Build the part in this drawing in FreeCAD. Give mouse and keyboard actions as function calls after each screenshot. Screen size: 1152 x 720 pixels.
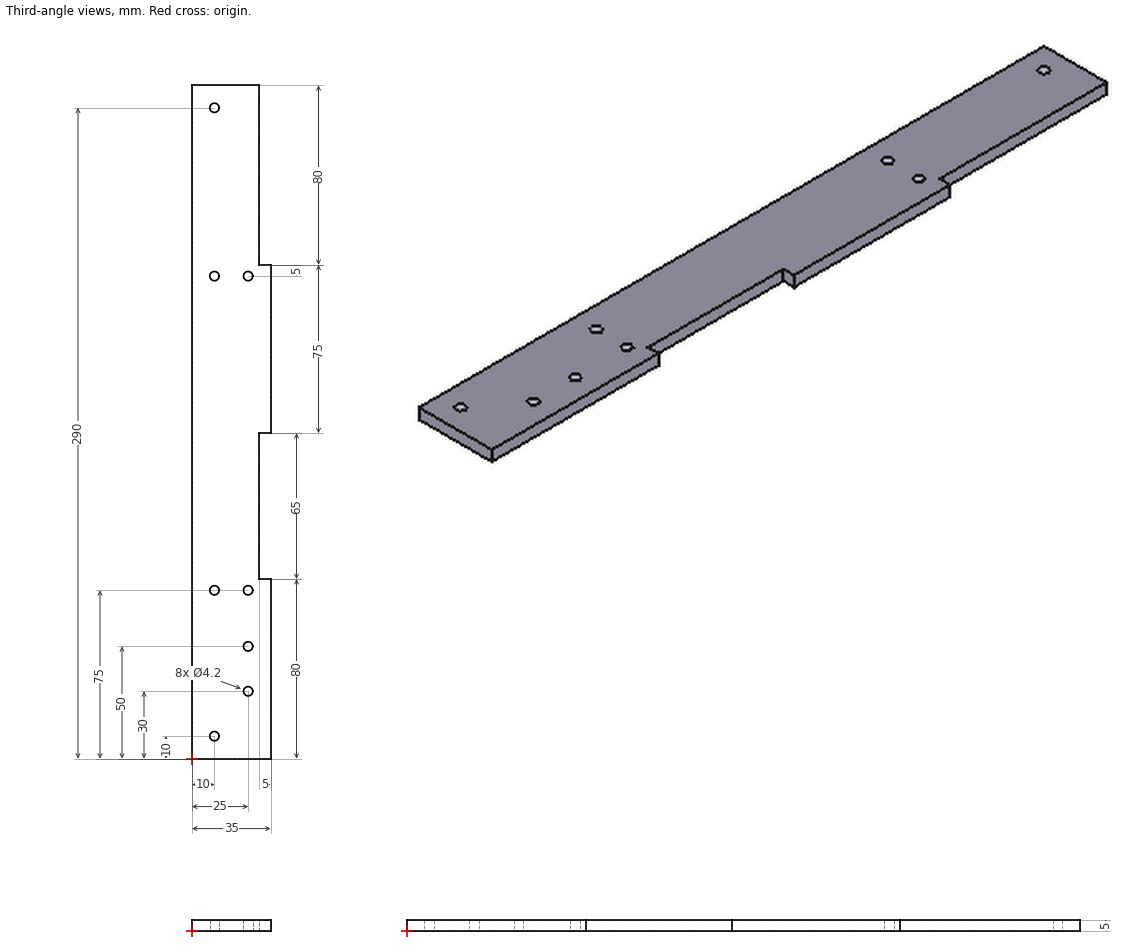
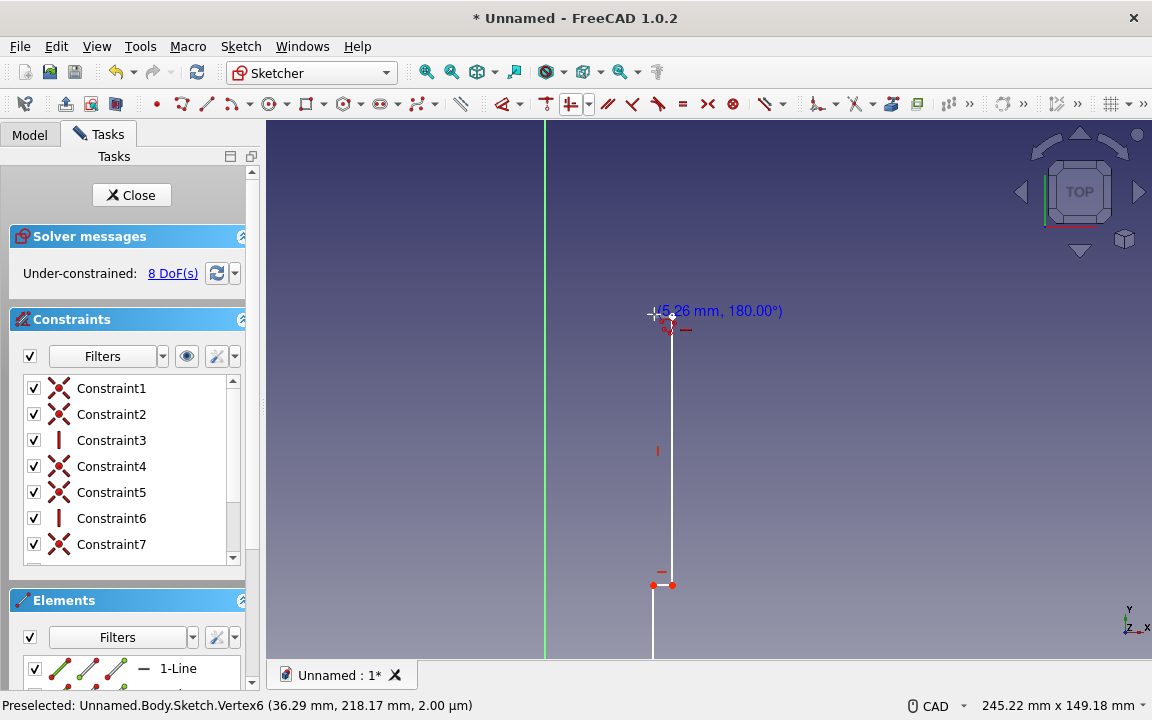
click(653, 313)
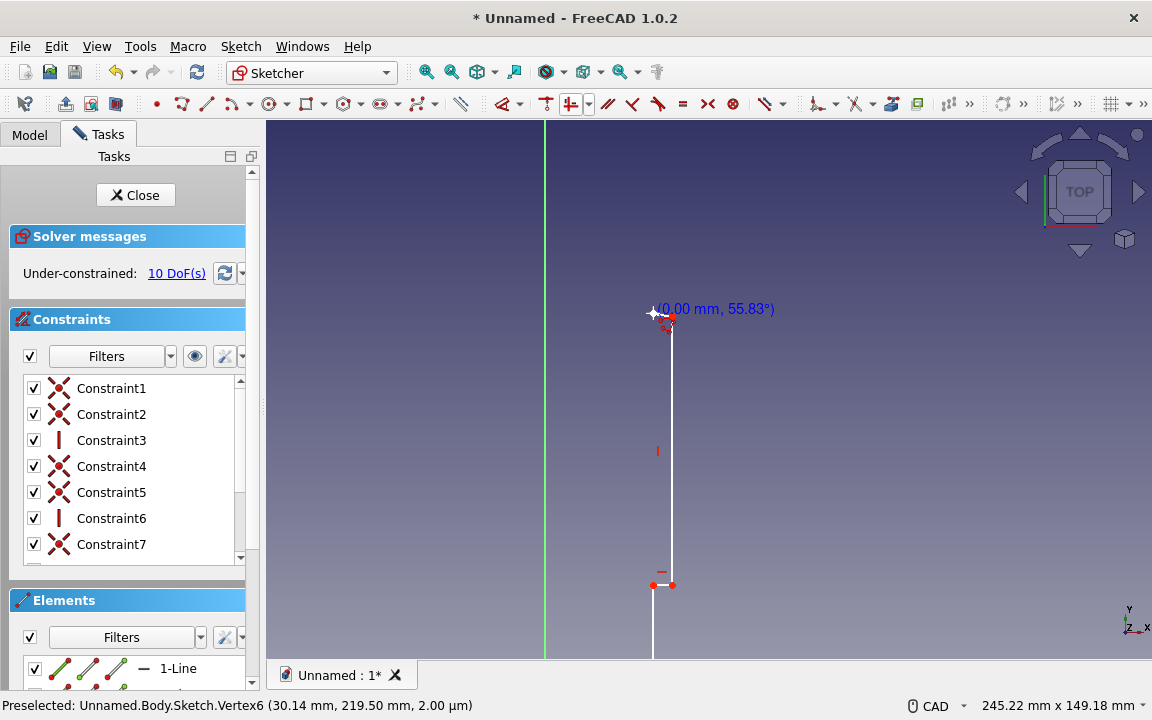
scroll(654, 313, down, 6)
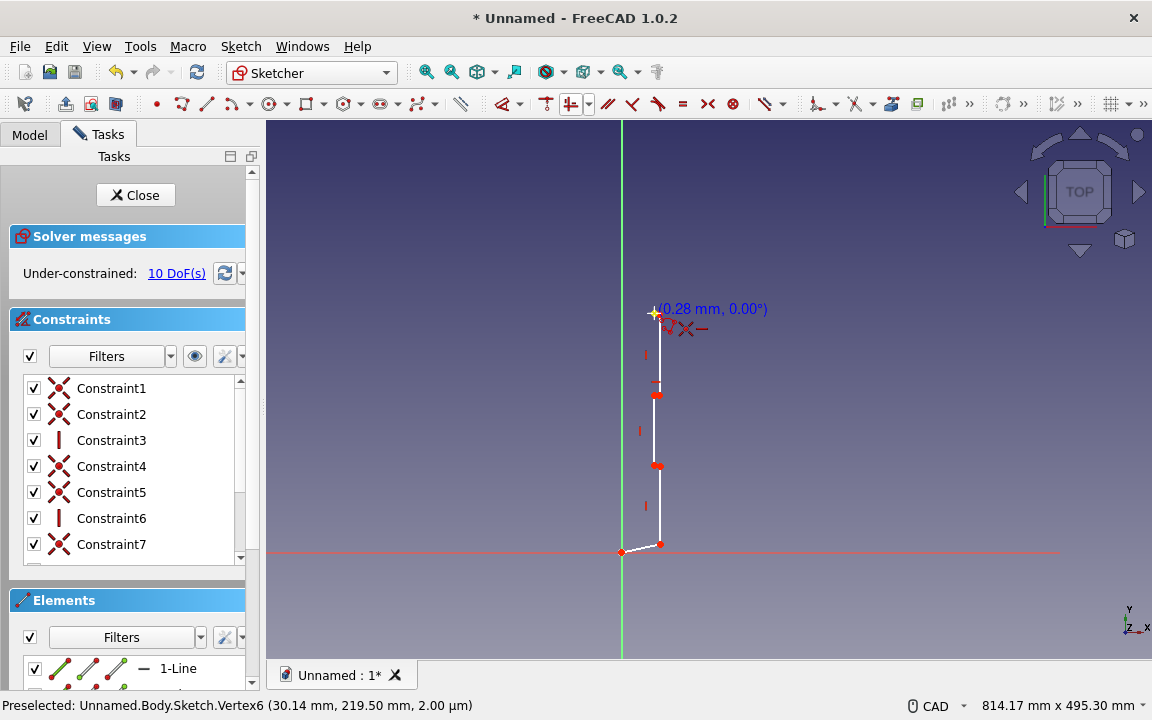
click(654, 226)
click(631, 226)
click(622, 553)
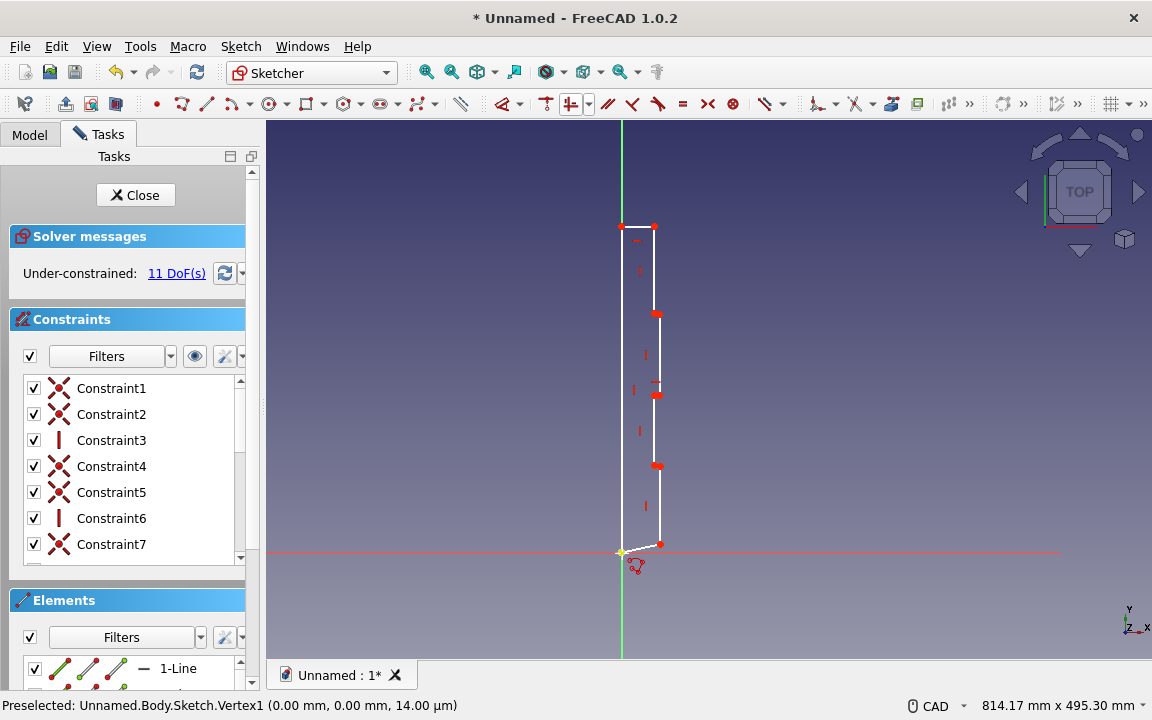
click(268, 104)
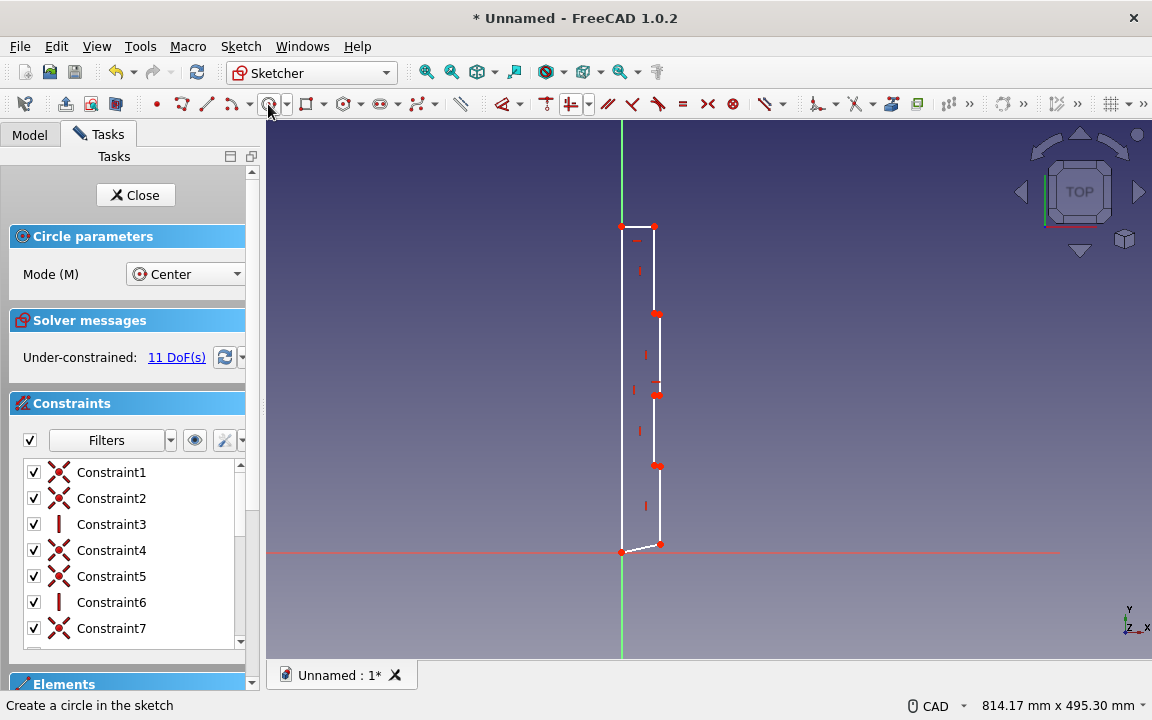
scroll(649, 520, up, 12)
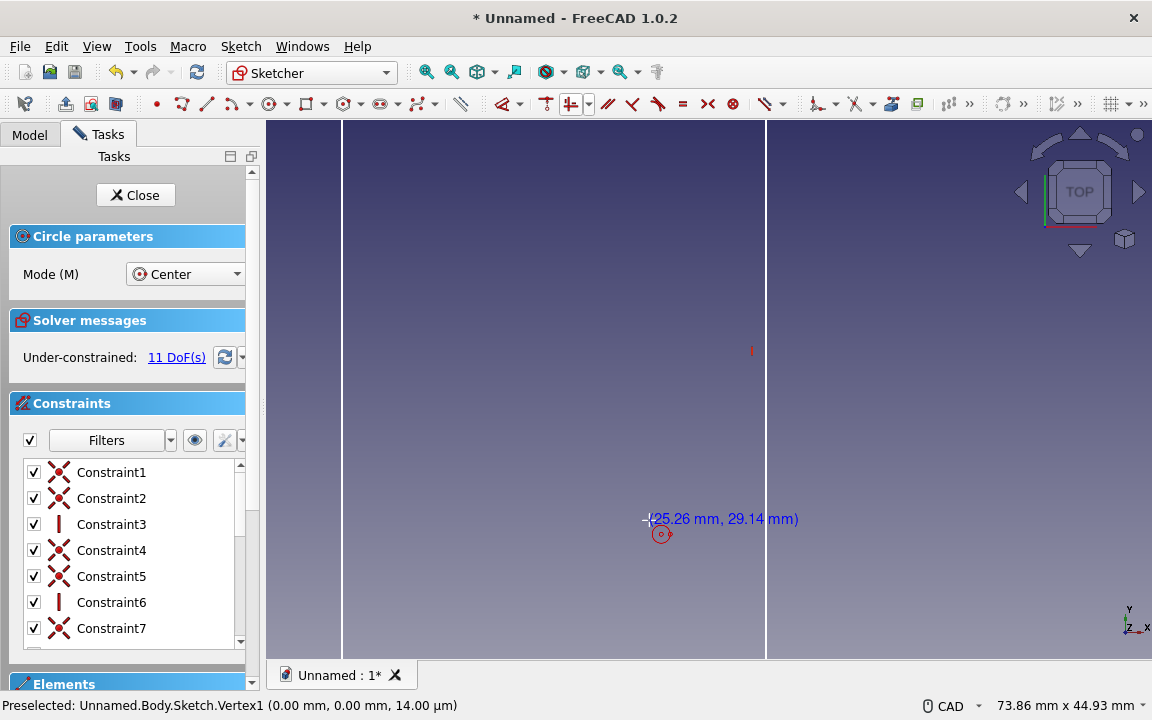
scroll(649, 521, down, 12)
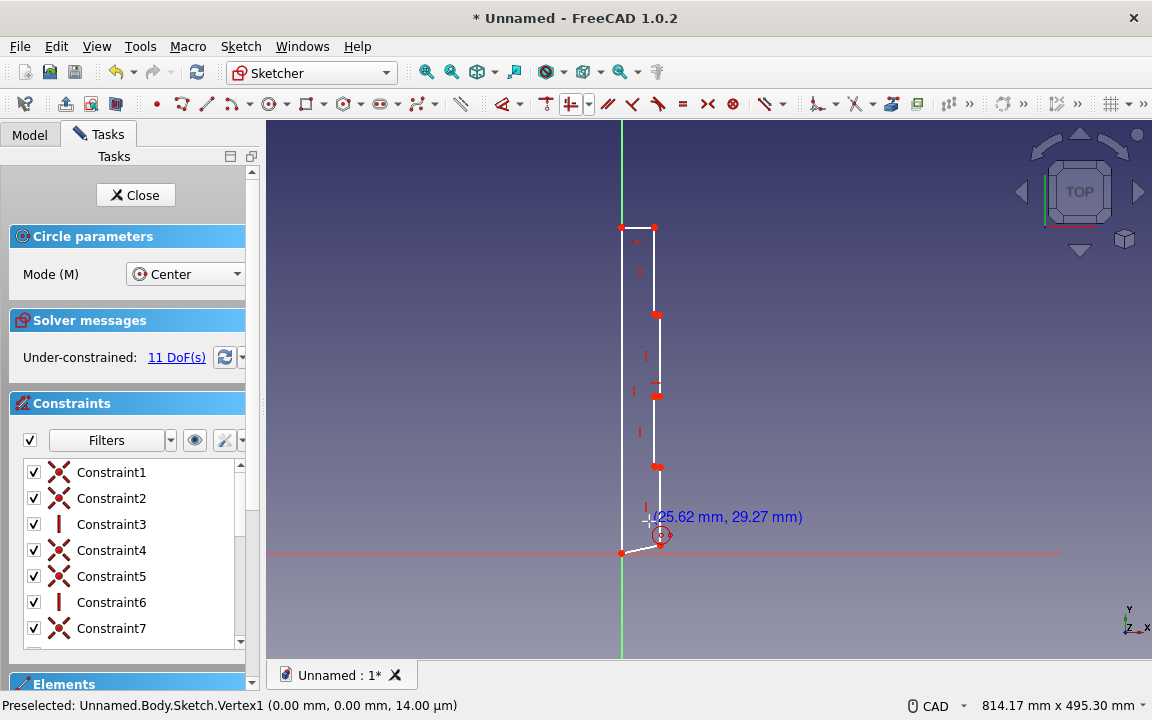
scroll(649, 521, up, 2)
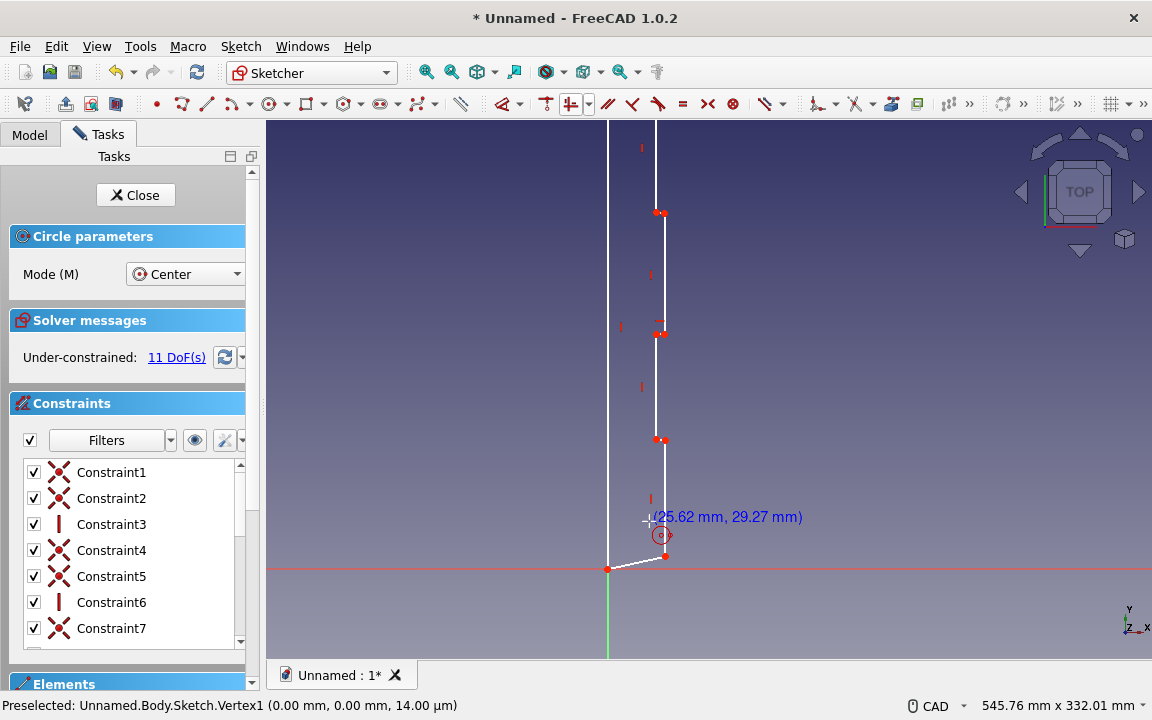
click(648, 521)
move(646, 518)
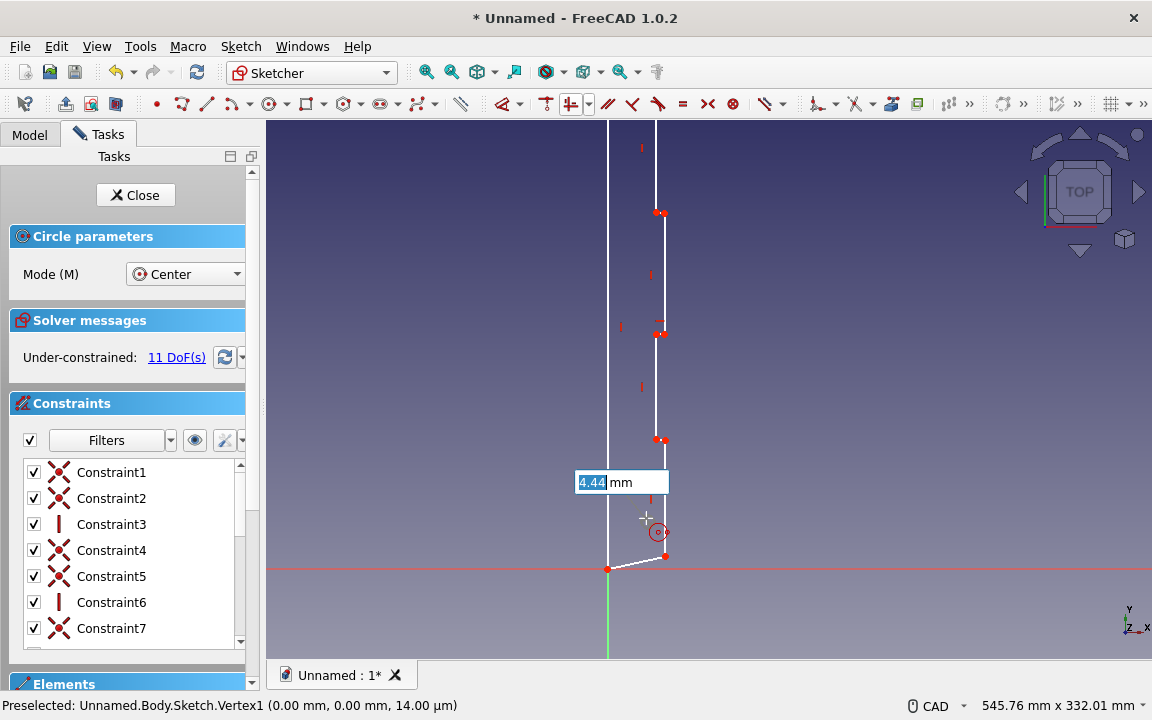
text(4.2)
key(Return)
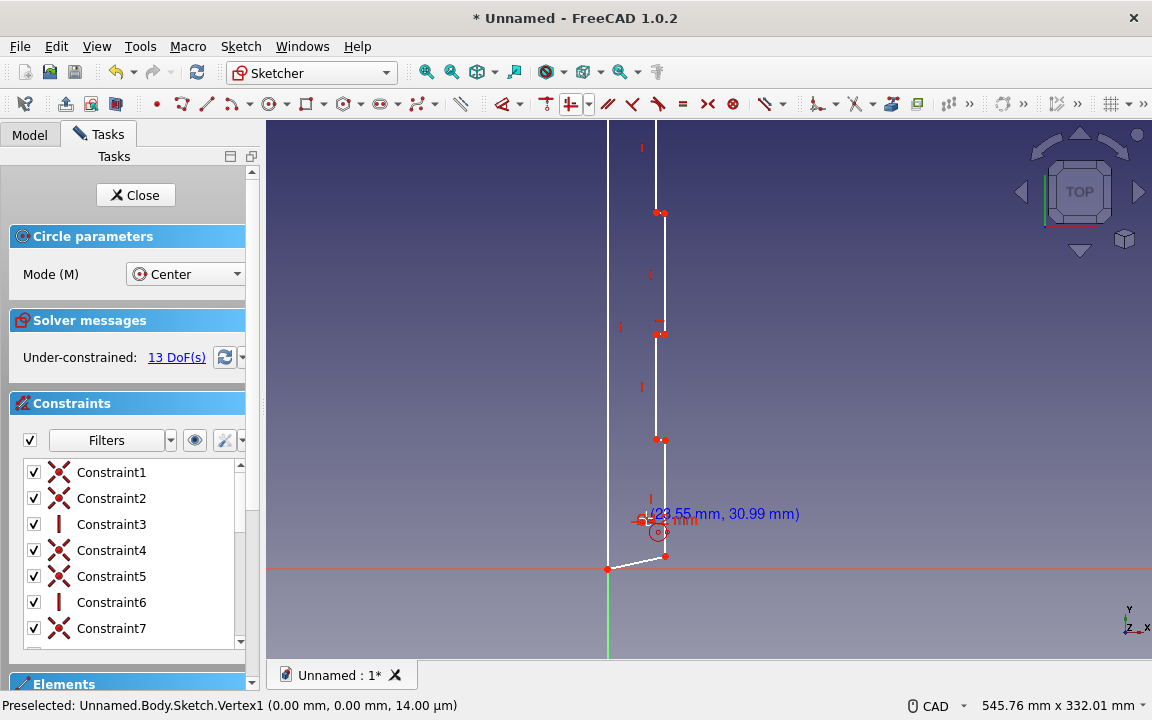
scroll(648, 488, up, 10)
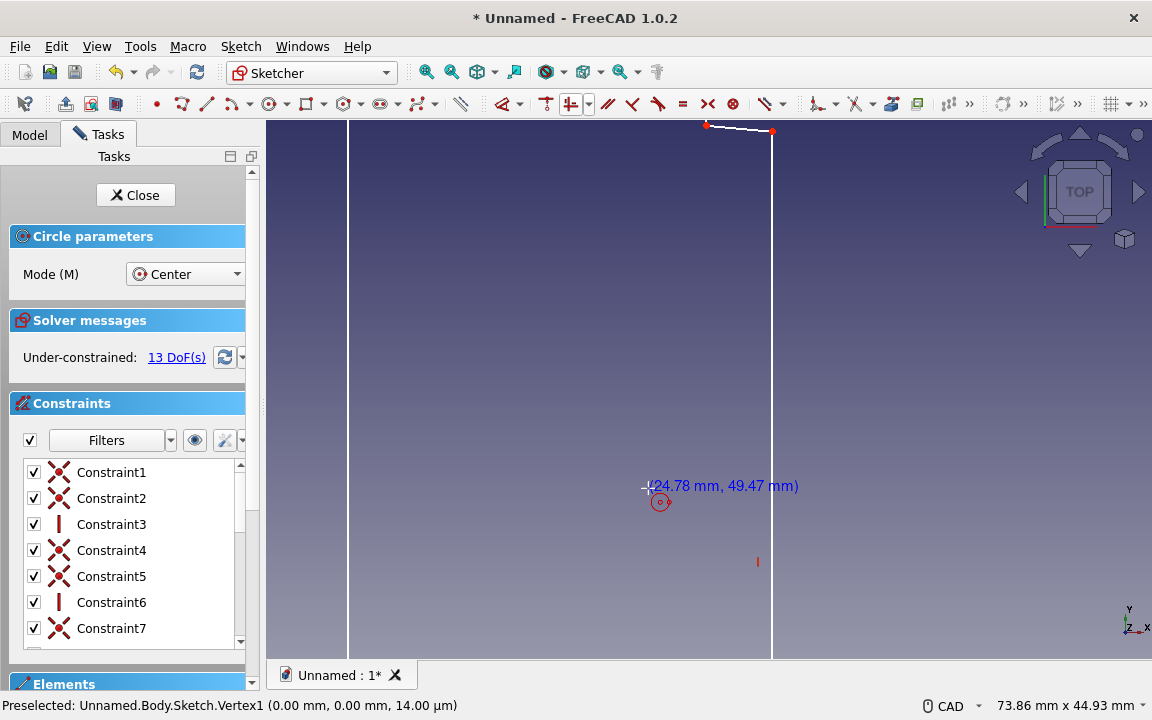
scroll(649, 500, down, 12)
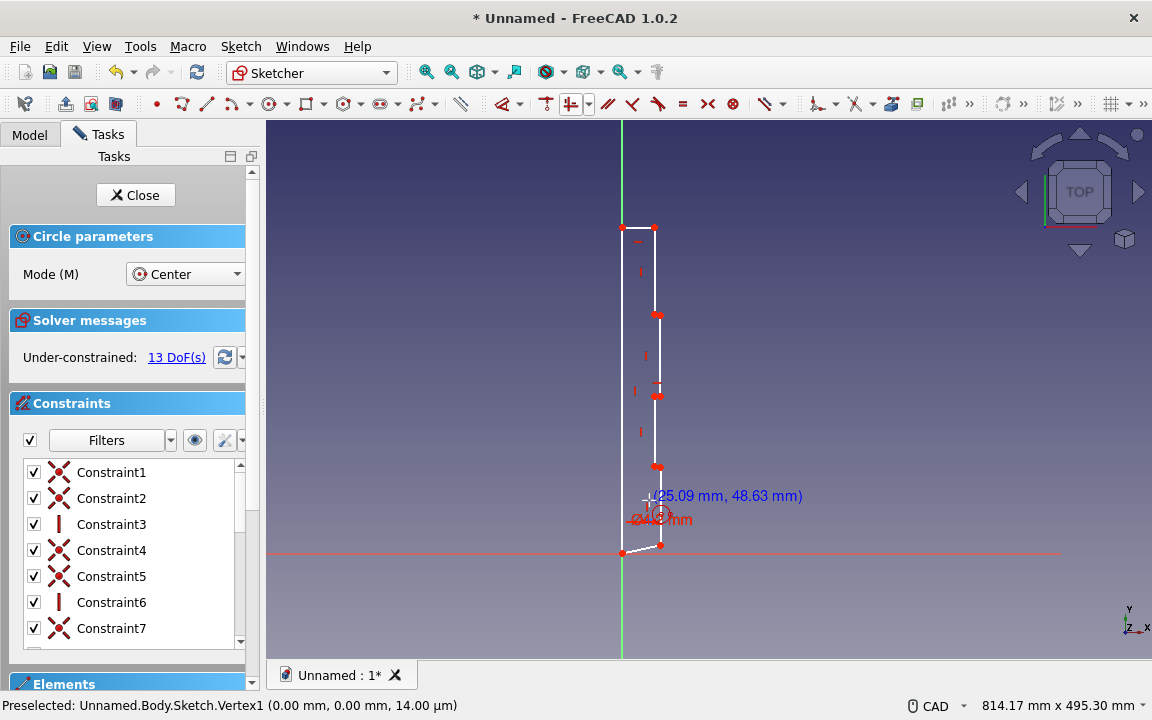
scroll(649, 499, up, 2)